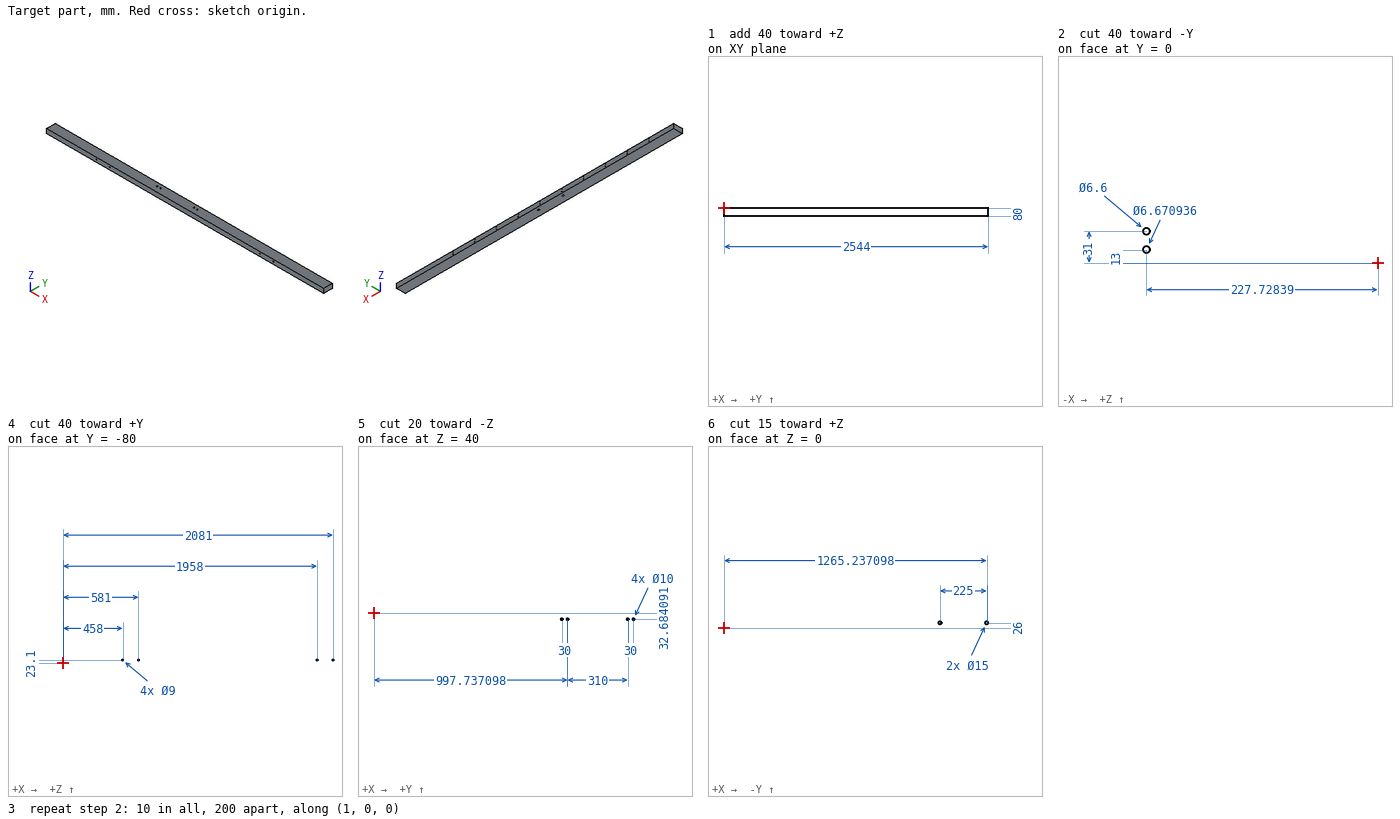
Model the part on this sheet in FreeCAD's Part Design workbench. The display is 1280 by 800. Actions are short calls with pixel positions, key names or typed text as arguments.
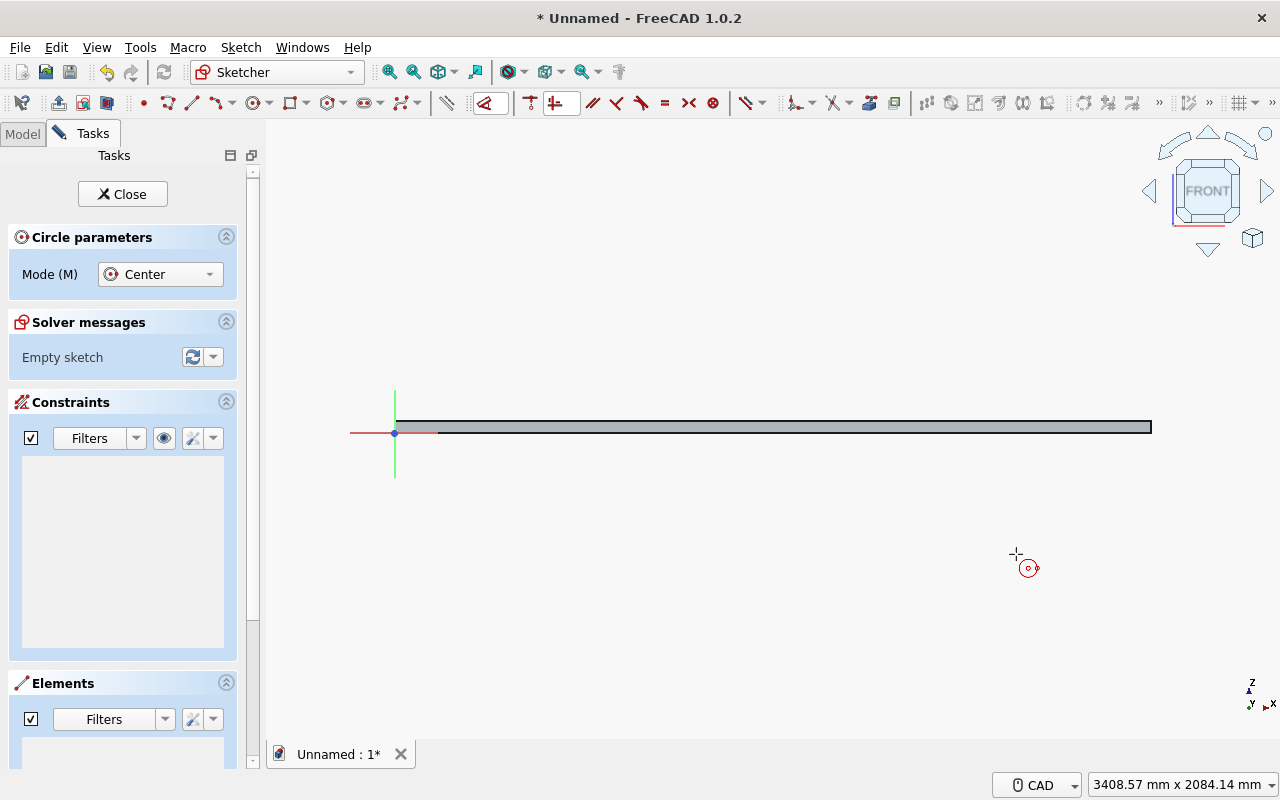
scroll(531, 426, up, 15)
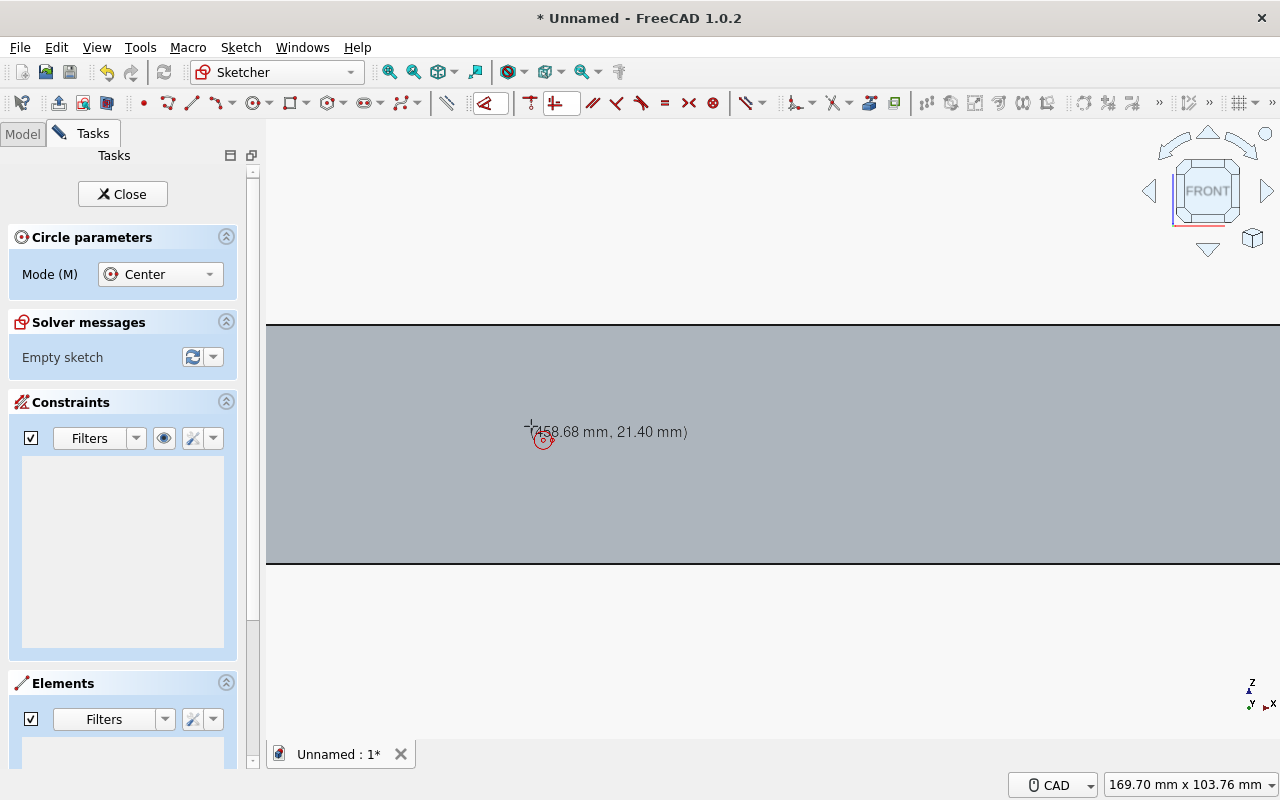
scroll(531, 426, down, 15)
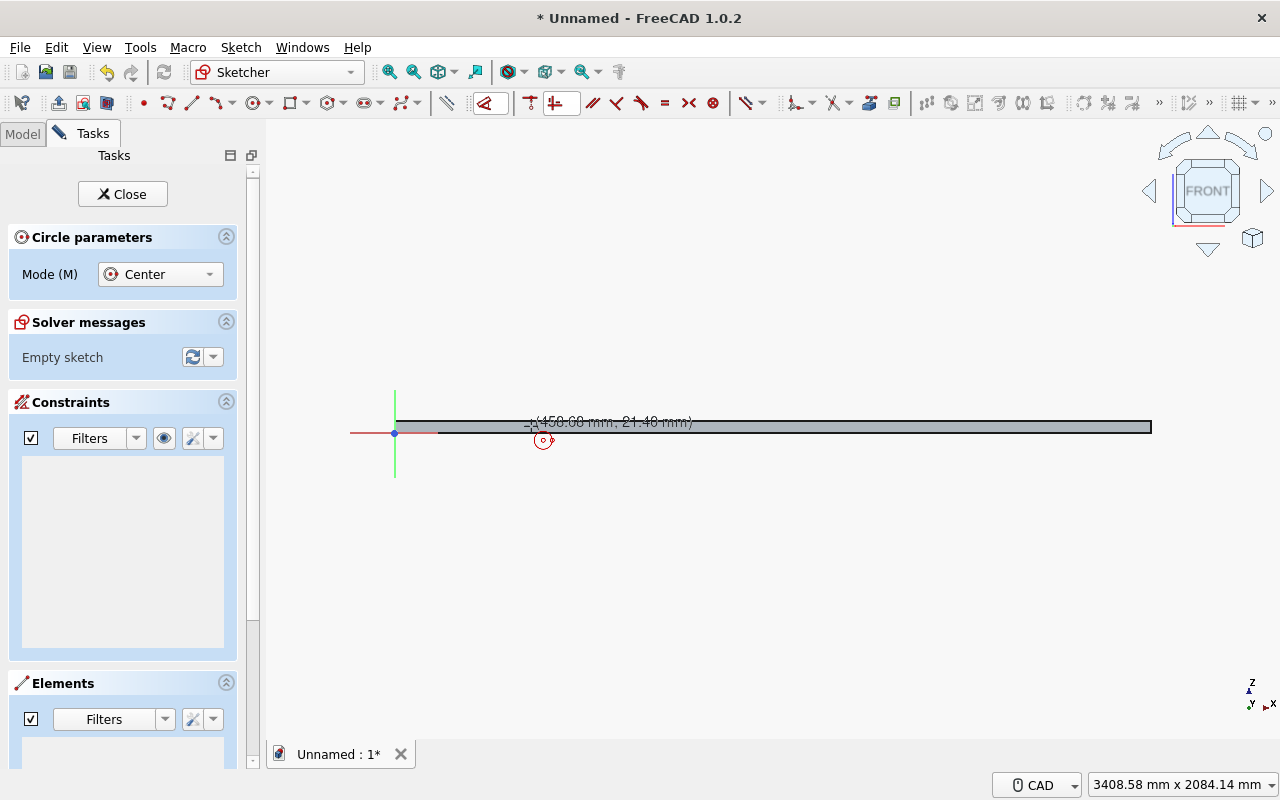
scroll(531, 426, up, 5)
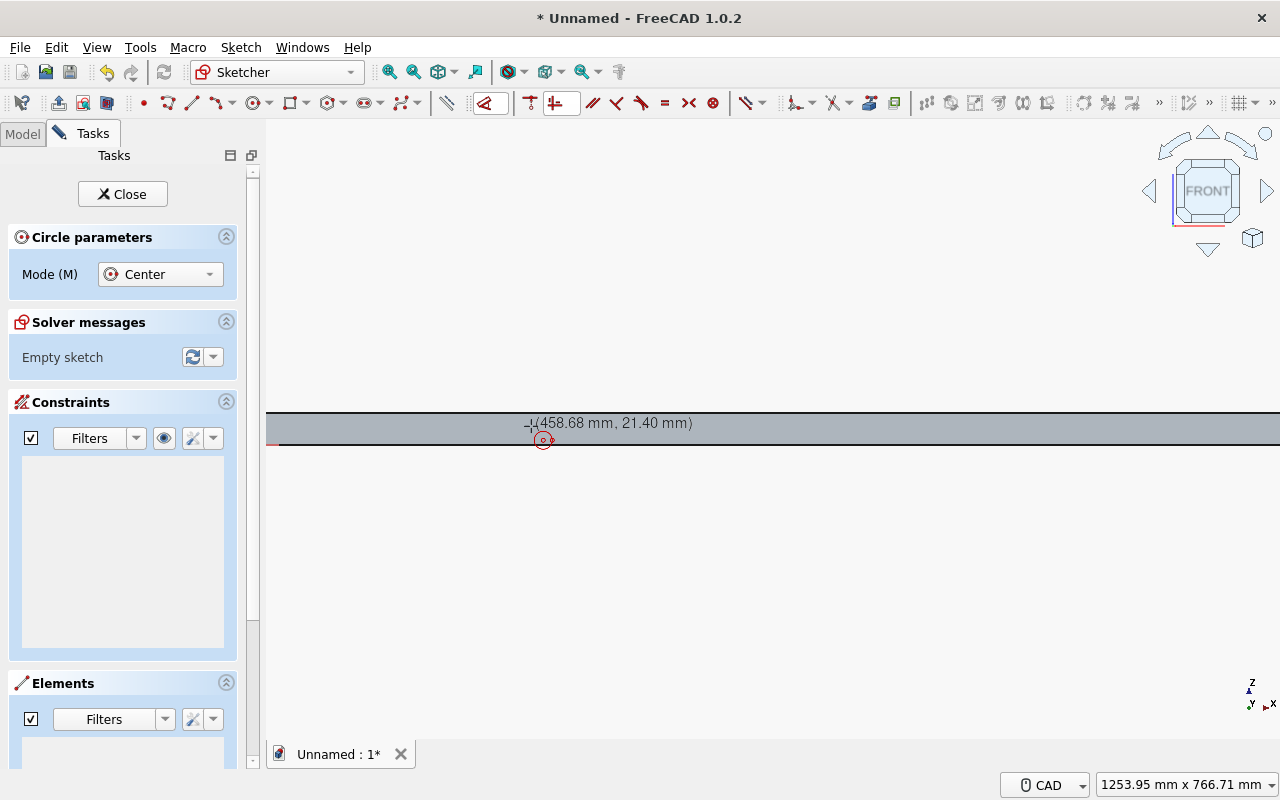
click(530, 426)
move(533, 424)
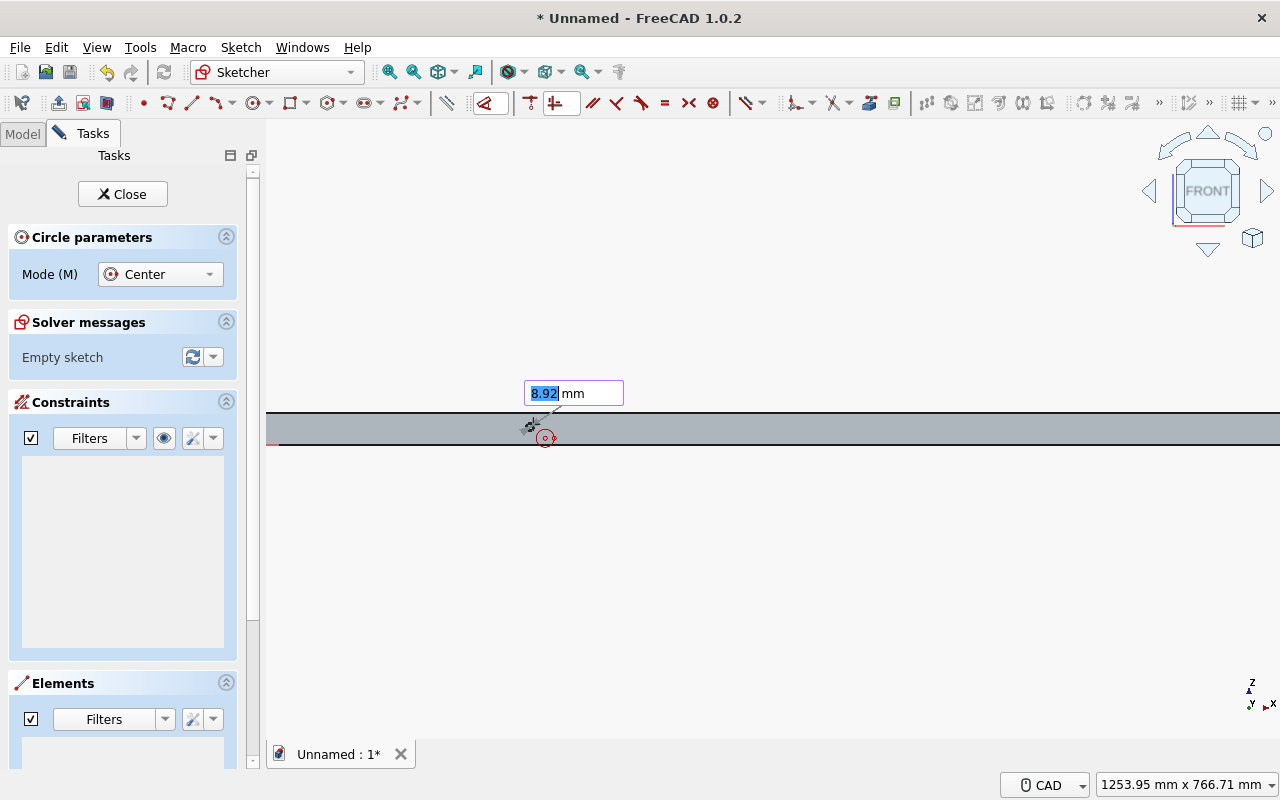
text(9)
key(Return)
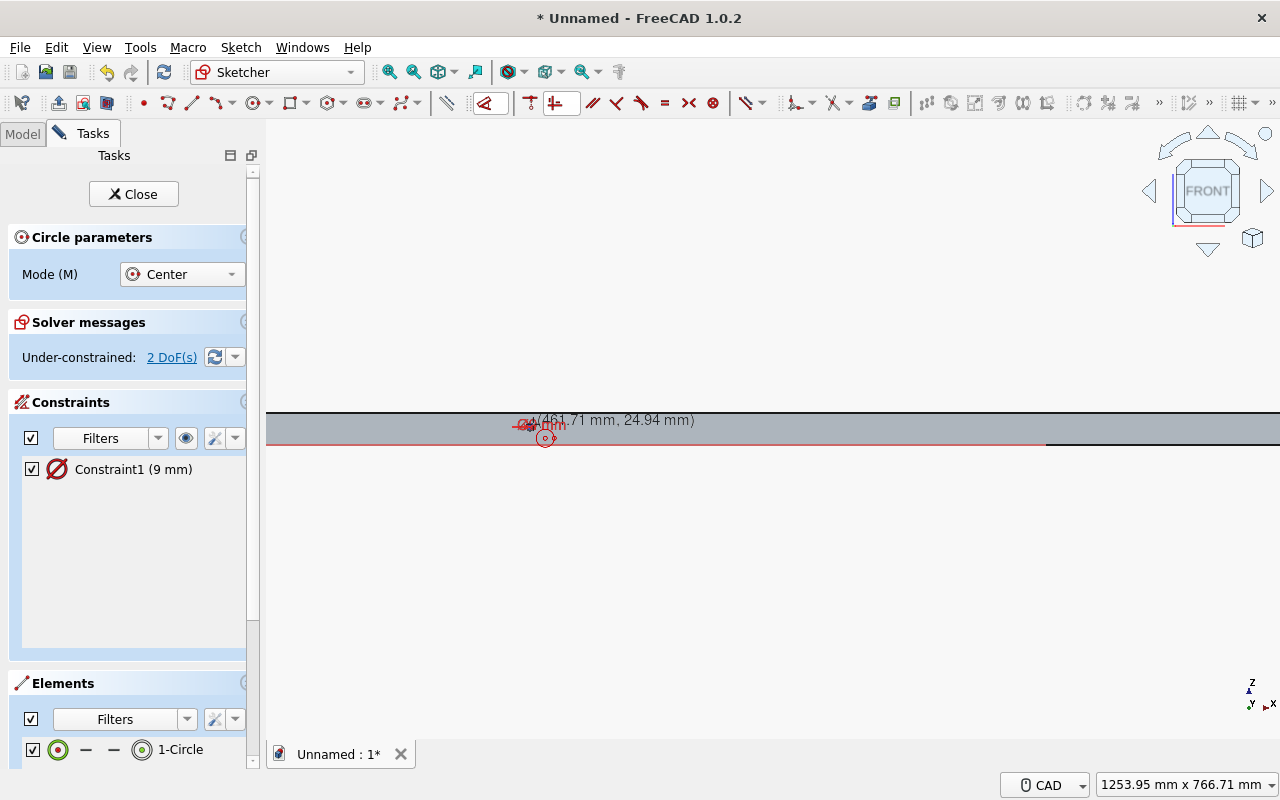
scroll(629, 426, up, 10)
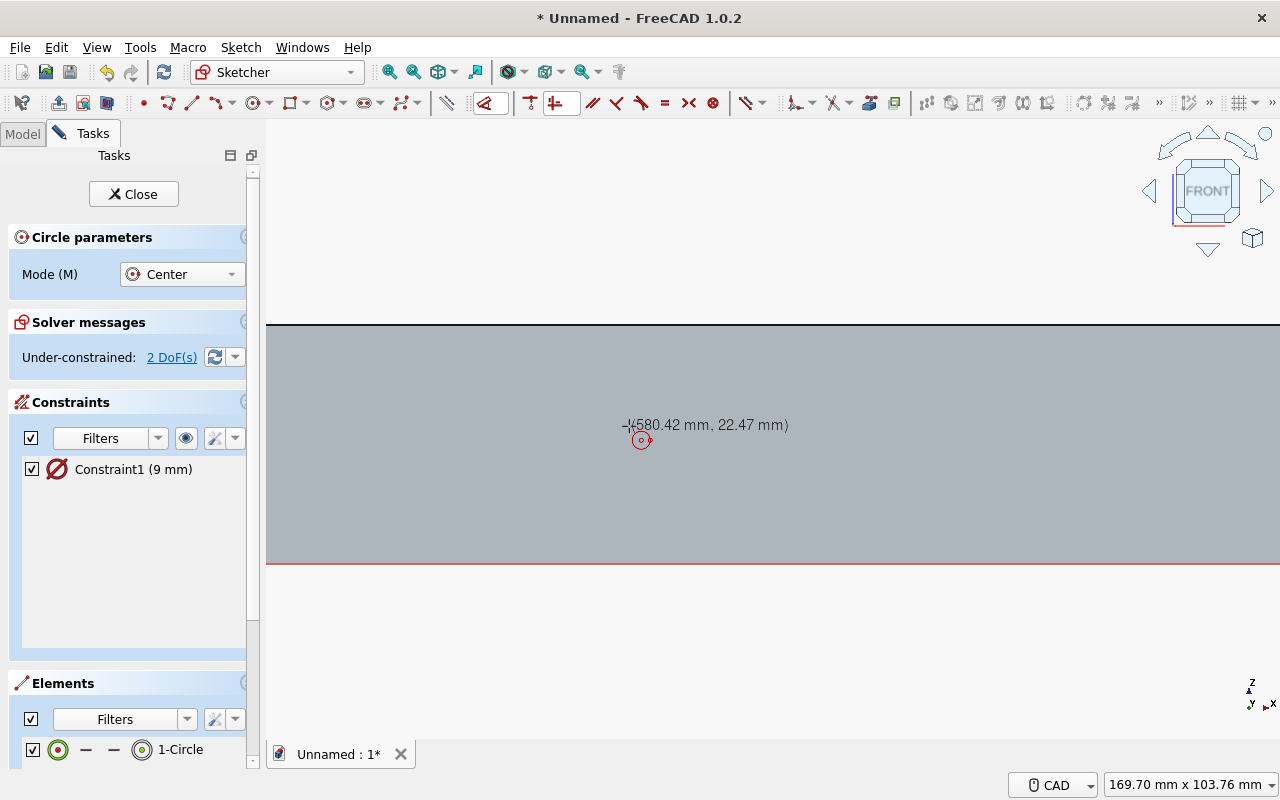
scroll(564, 426, down, 15)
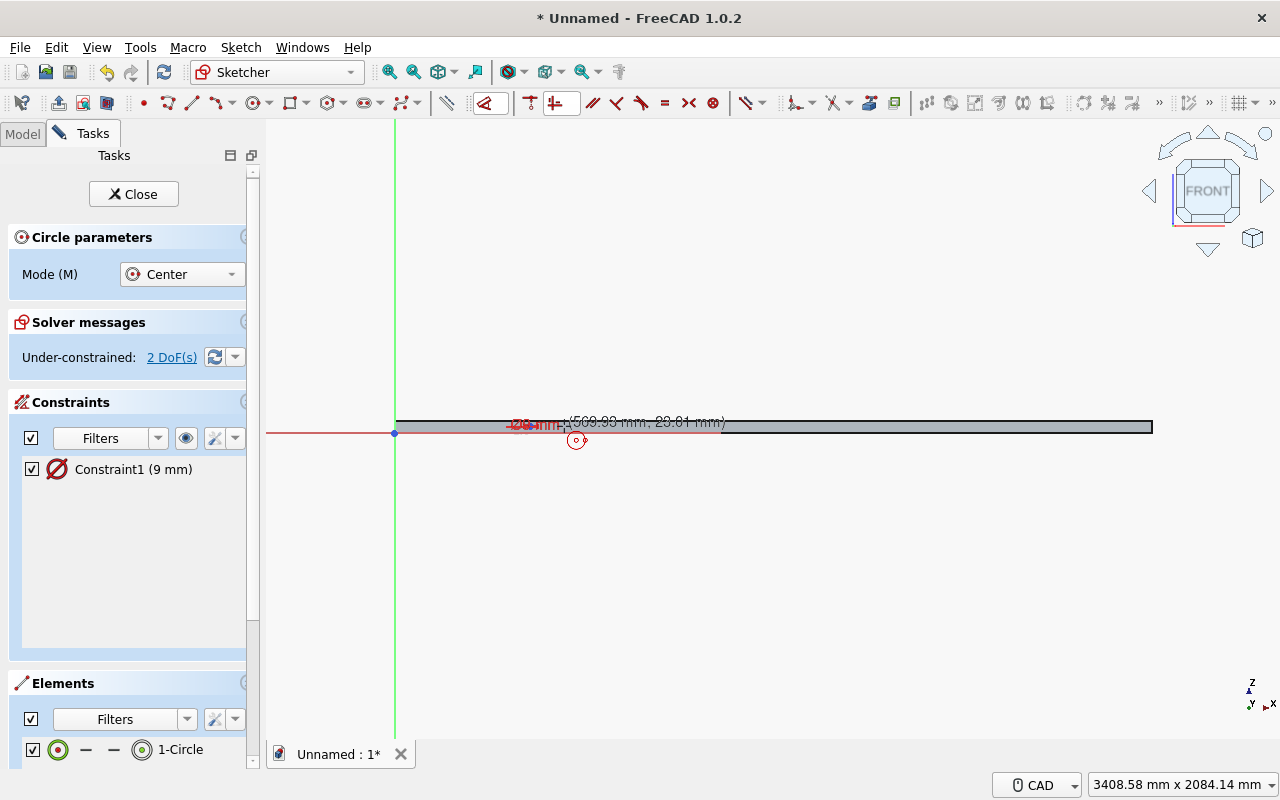
scroll(568, 426, up, 5)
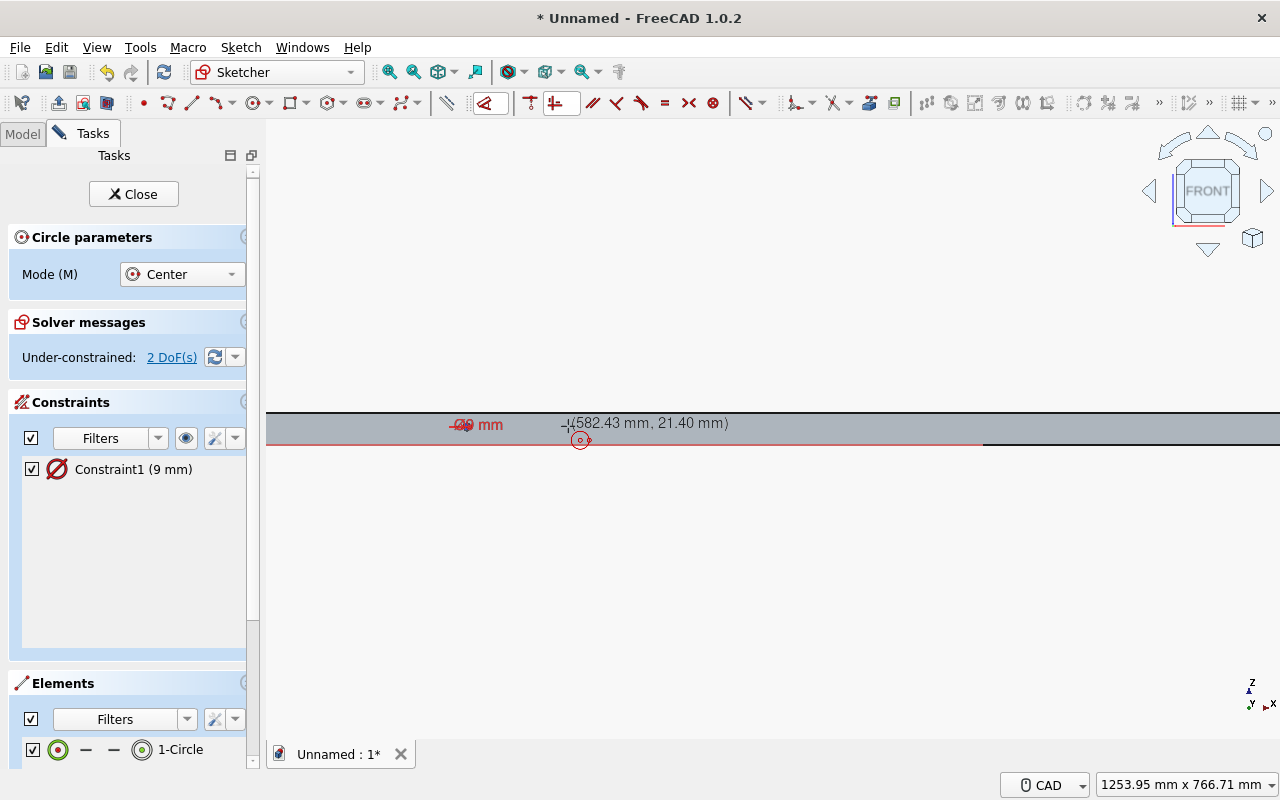
click(566, 426)
move(569, 424)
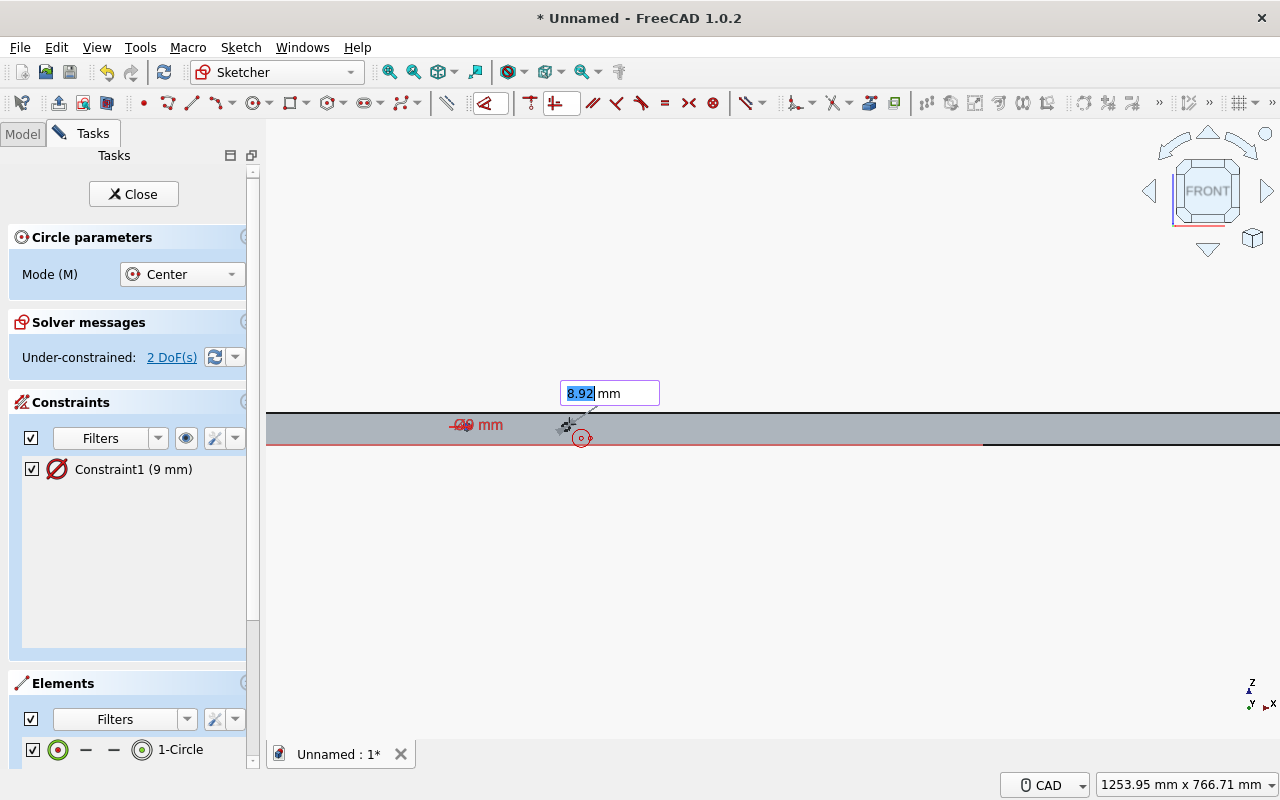
text(9)
key(Return)